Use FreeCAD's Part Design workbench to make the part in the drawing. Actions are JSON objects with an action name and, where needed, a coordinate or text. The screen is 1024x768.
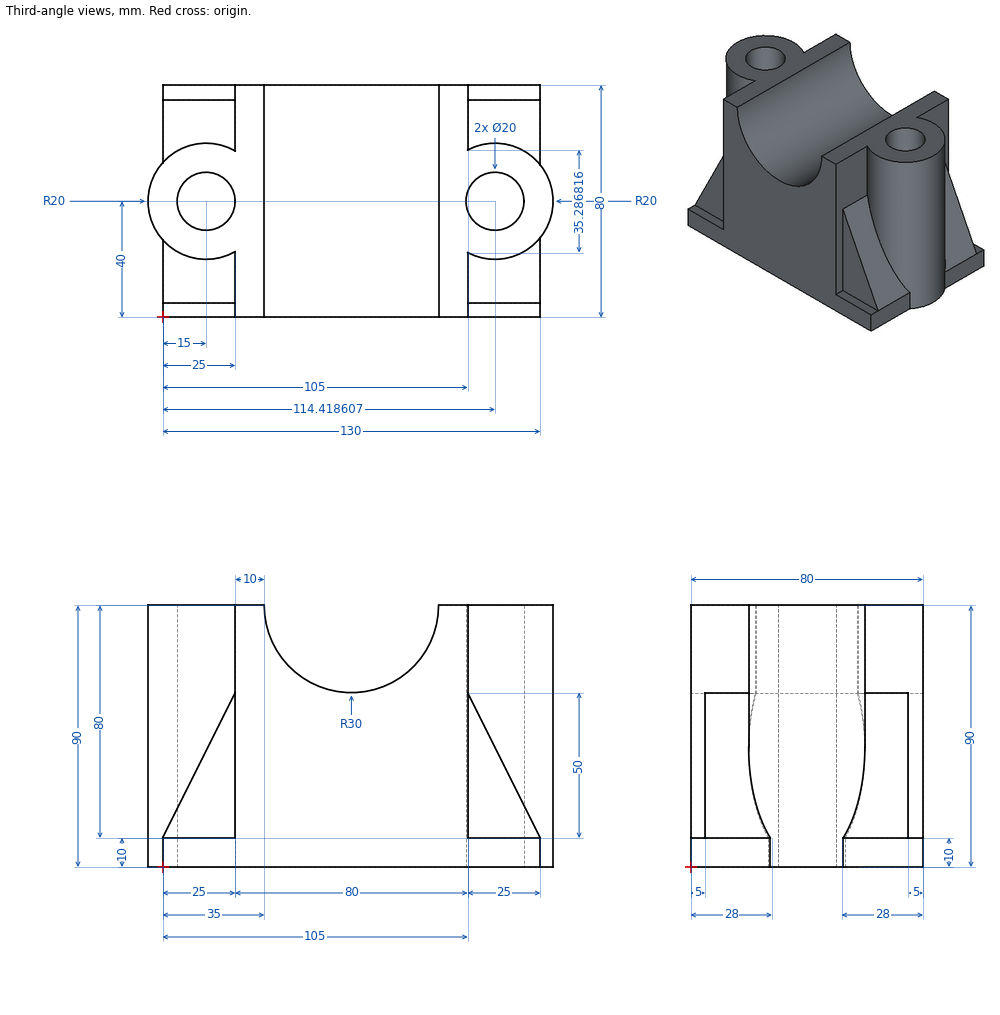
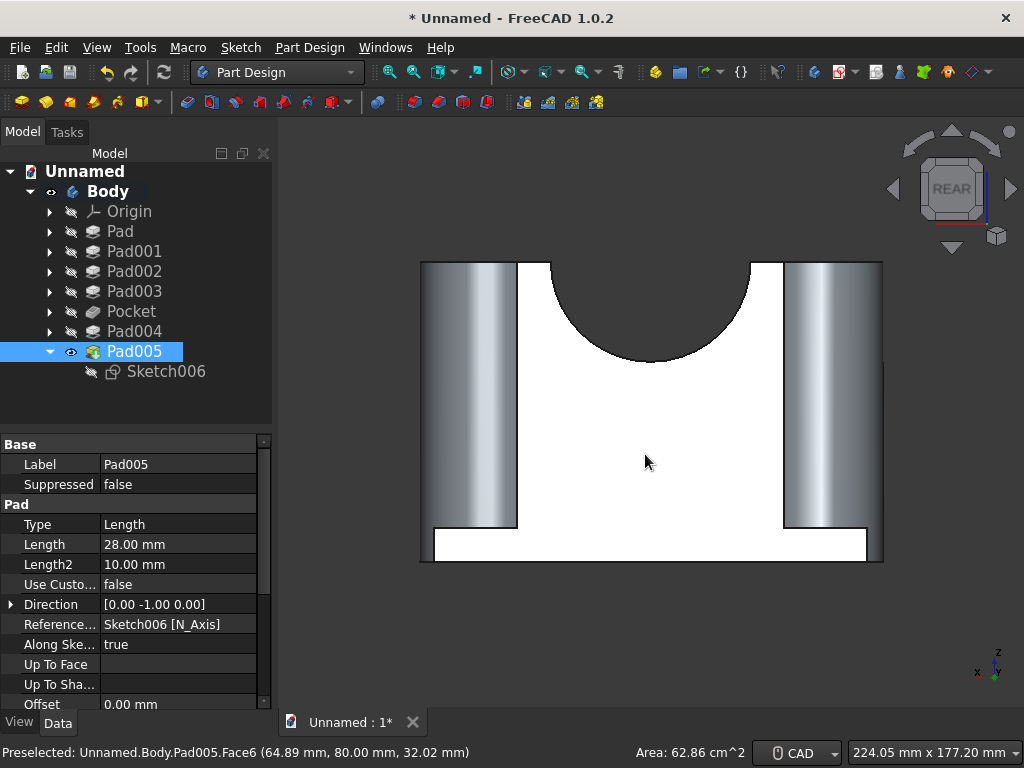
{"action": "left_click", "coordinate": [840, 72]}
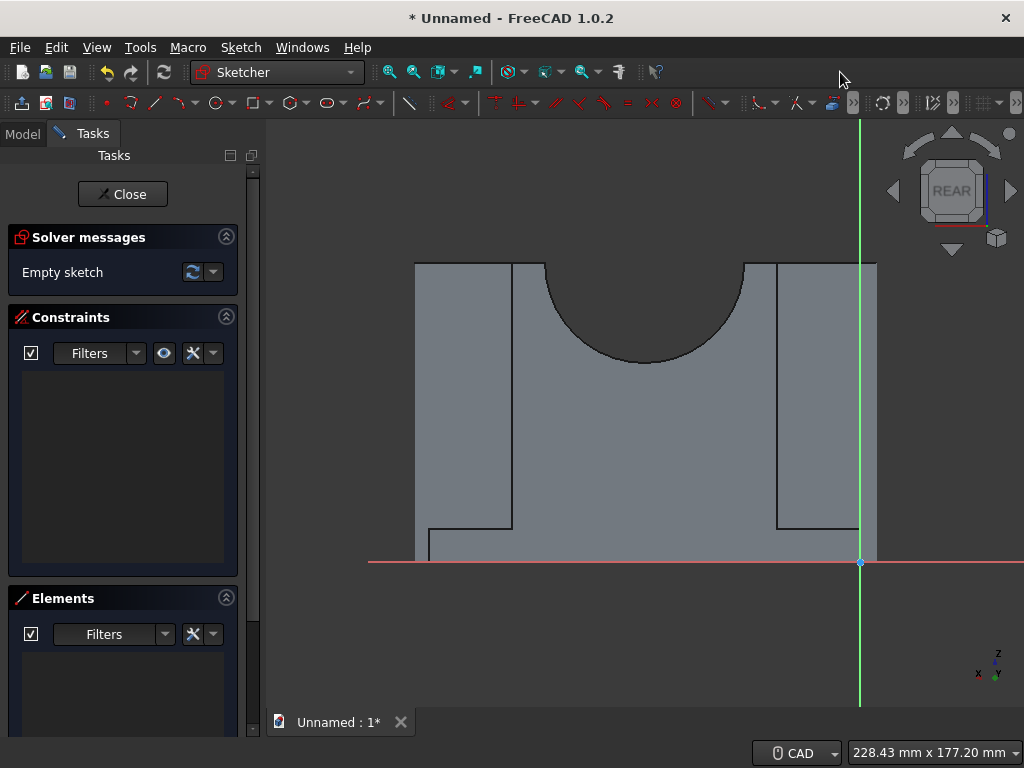
{"action": "scroll", "coordinate": [294, 189], "scroll_direction": "down", "scroll_amount": 1}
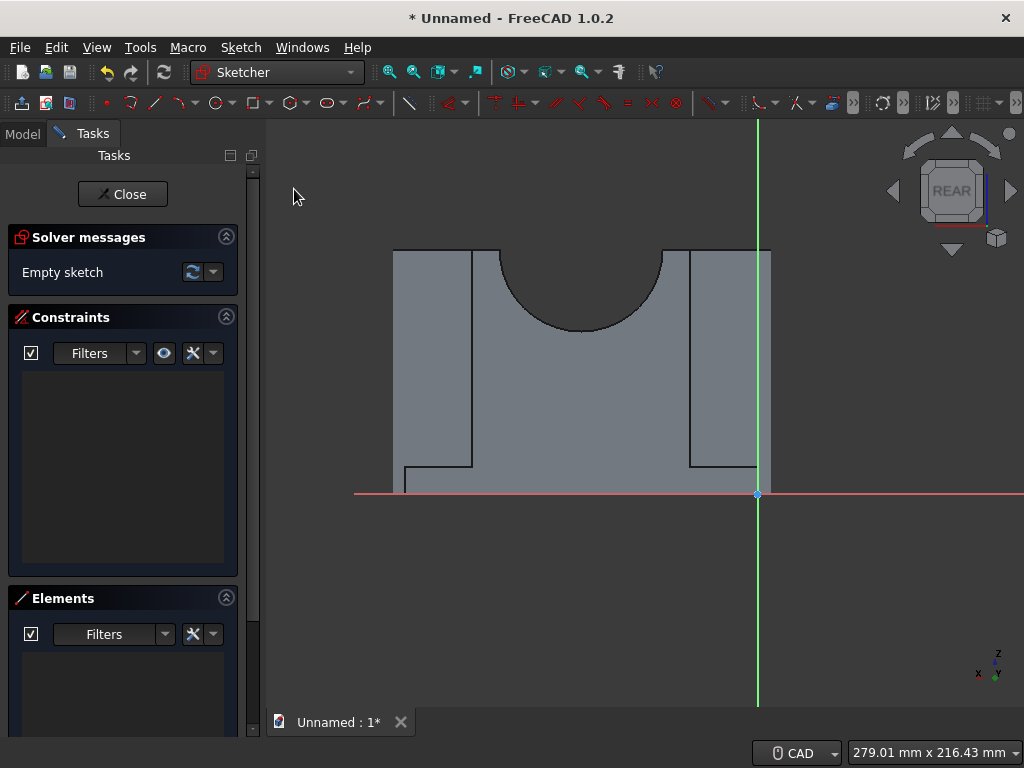
{"action": "left_click", "coordinate": [132, 104]}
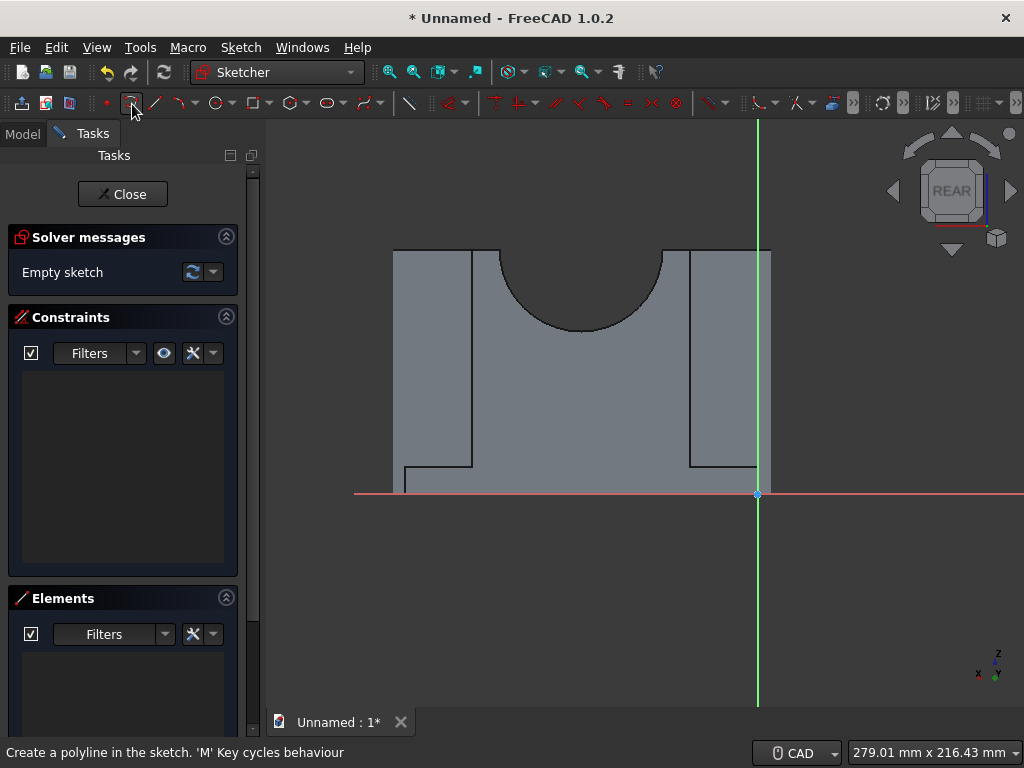
{"action": "left_click", "coordinate": [472, 467]}
{"action": "left_click", "coordinate": [472, 331]}
{"action": "left_click", "coordinate": [405, 467]}
{"action": "left_click", "coordinate": [472, 468]}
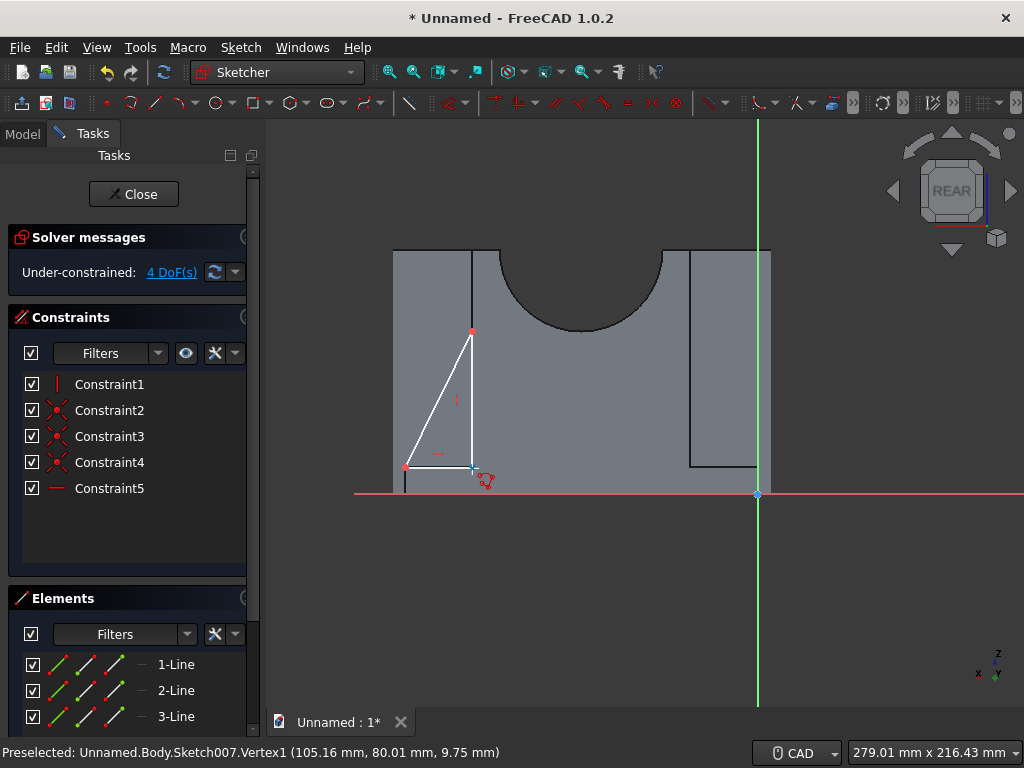
{"action": "left_click", "coordinate": [758, 467]}
{"action": "left_click", "coordinate": [690, 331]}
{"action": "left_click", "coordinate": [690, 467]}
{"action": "left_click", "coordinate": [758, 468]}
{"action": "key", "text": "Escape"}
{"action": "key", "text": "Escape"}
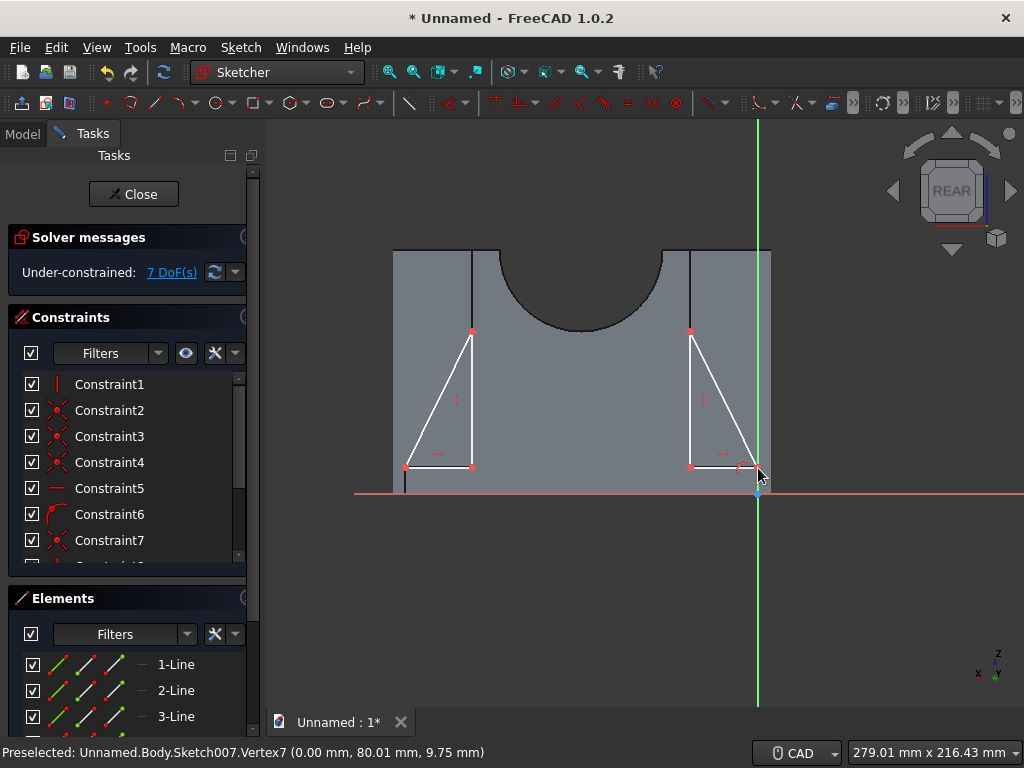
{"action": "left_click", "coordinate": [448, 104]}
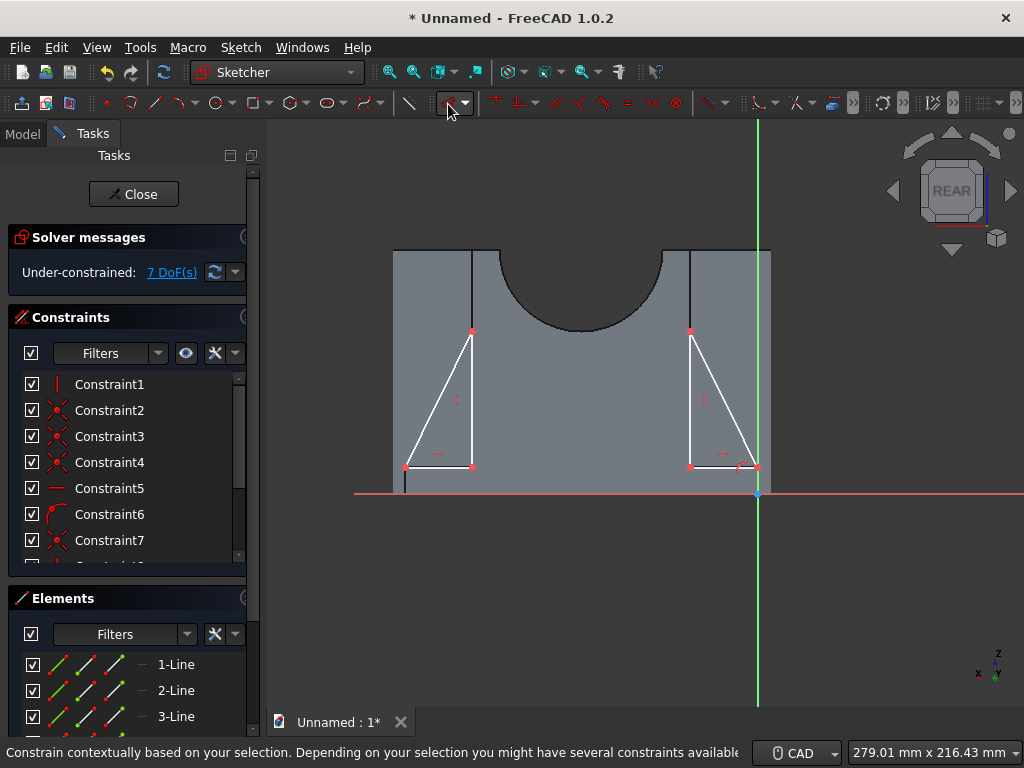
{"action": "left_click", "coordinate": [472, 427]}
{"action": "left_click", "coordinate": [438, 369]}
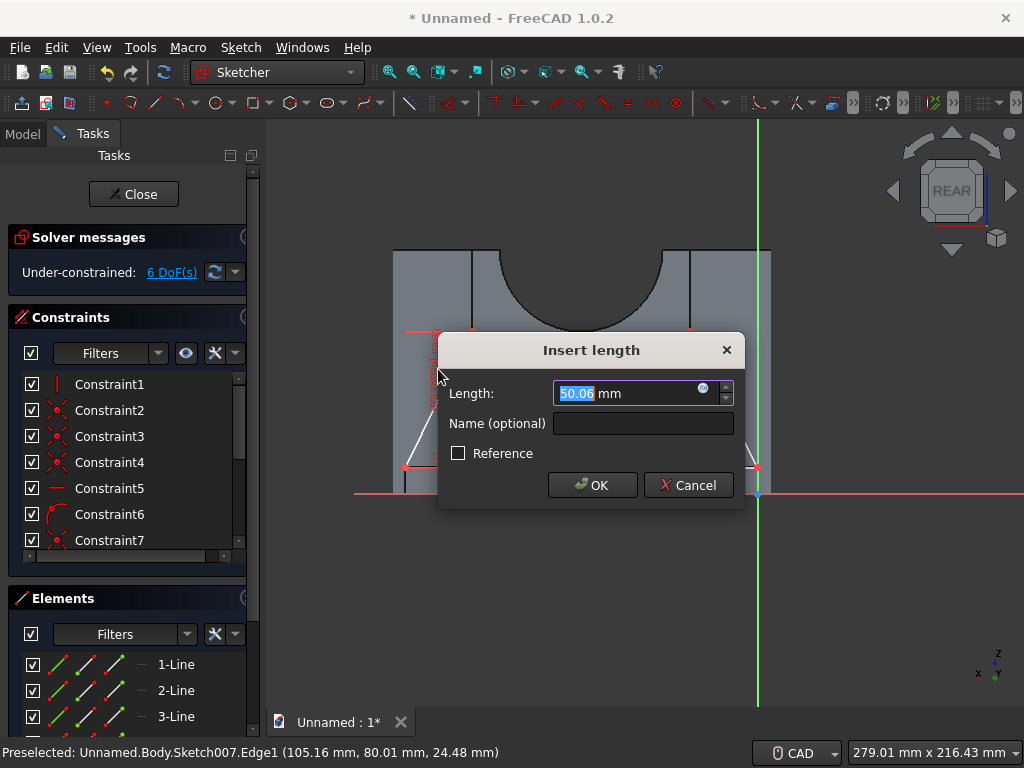
{"action": "type", "text": "50"}
{"action": "key", "text": "Return"}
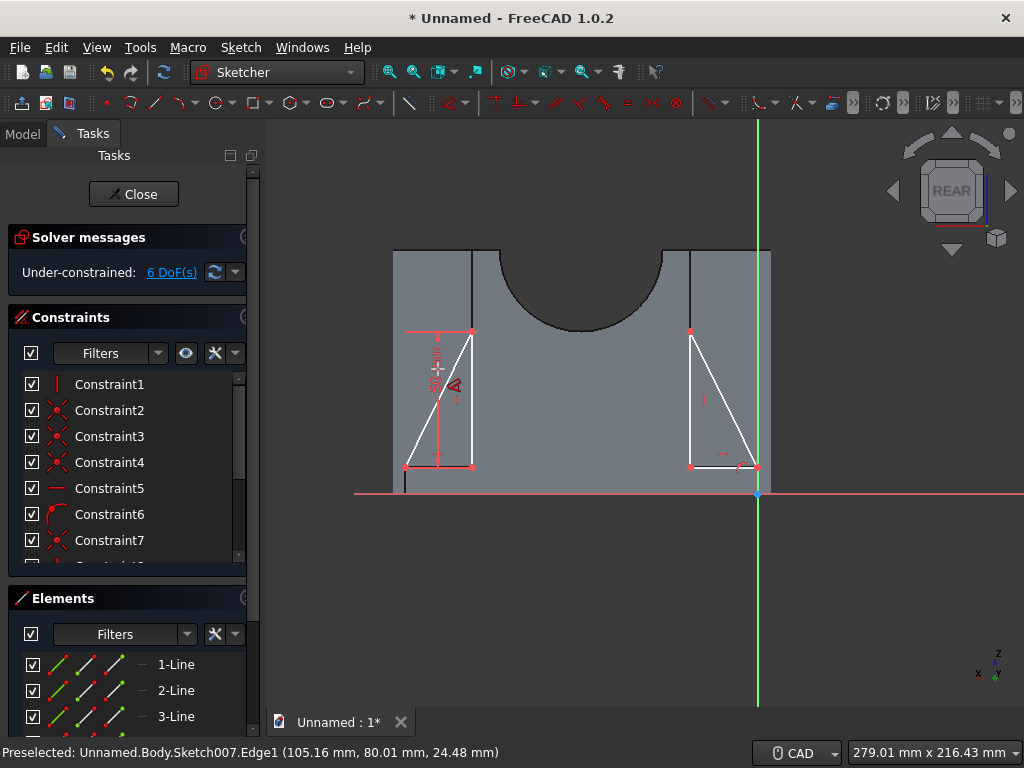
{"action": "left_click", "coordinate": [425, 468]}
{"action": "left_click", "coordinate": [439, 434]}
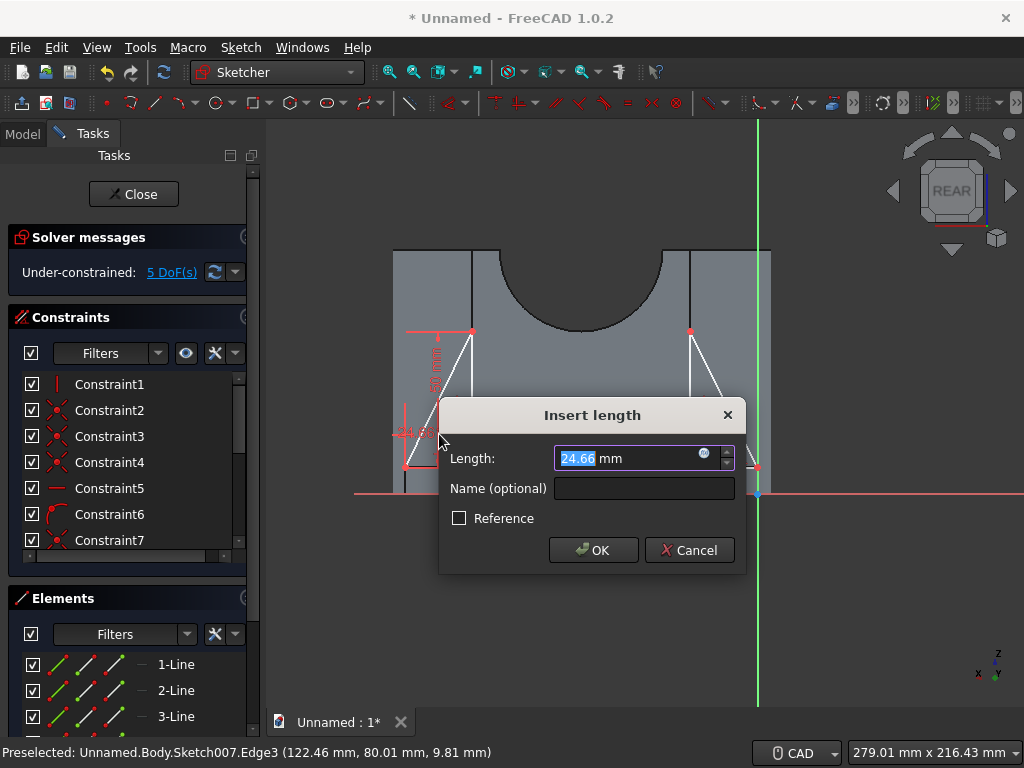
{"action": "type", "text": "25"}
{"action": "key", "text": "Return"}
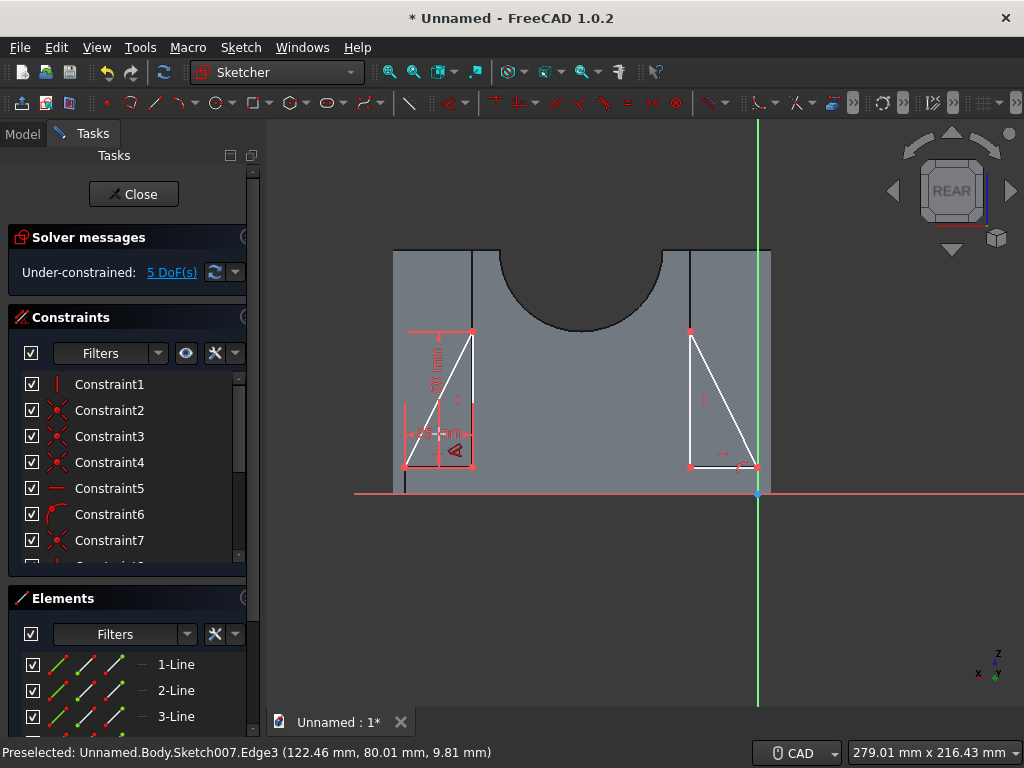
{"action": "left_click", "coordinate": [690, 373]}
{"action": "left_click", "coordinate": [724, 369]}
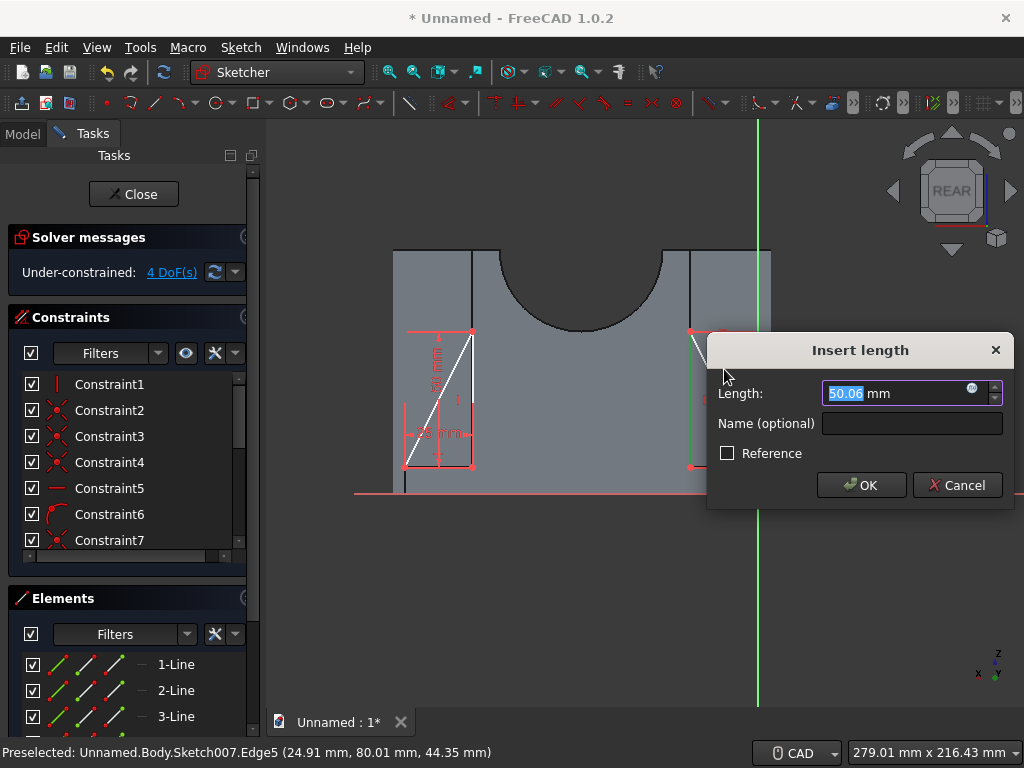
{"action": "type", "text": "50"}
{"action": "key", "text": "Return"}